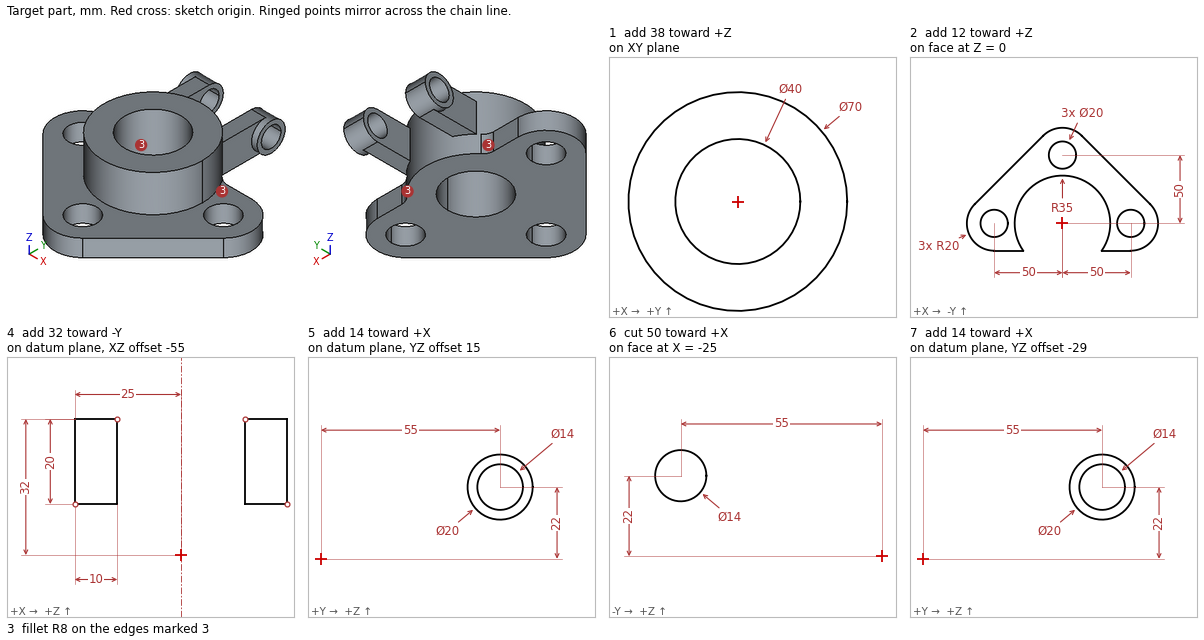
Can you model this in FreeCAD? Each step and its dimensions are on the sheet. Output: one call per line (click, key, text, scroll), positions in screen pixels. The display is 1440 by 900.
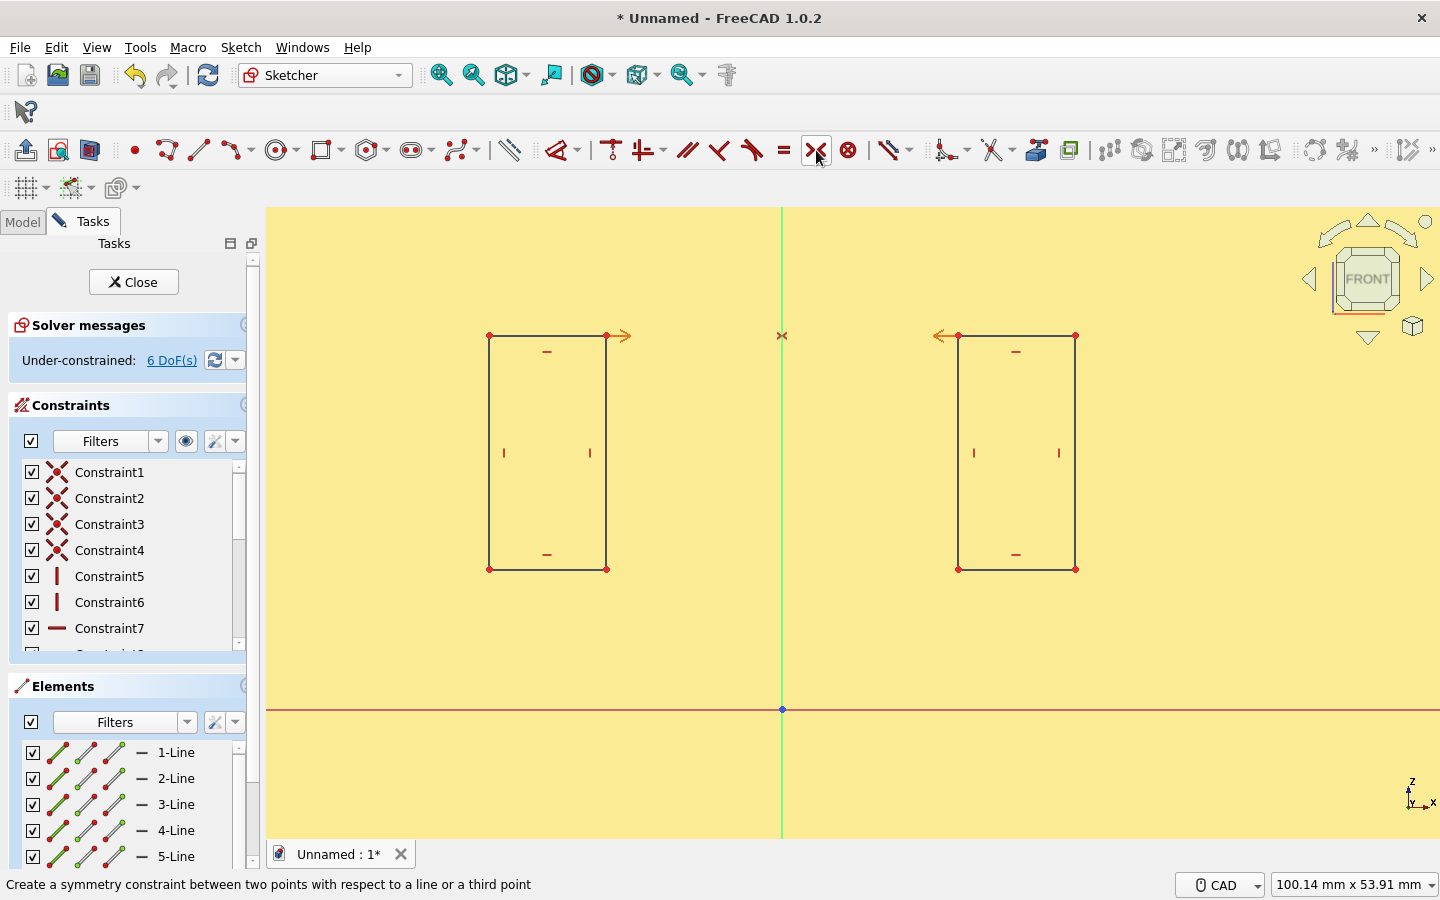
click(489, 570)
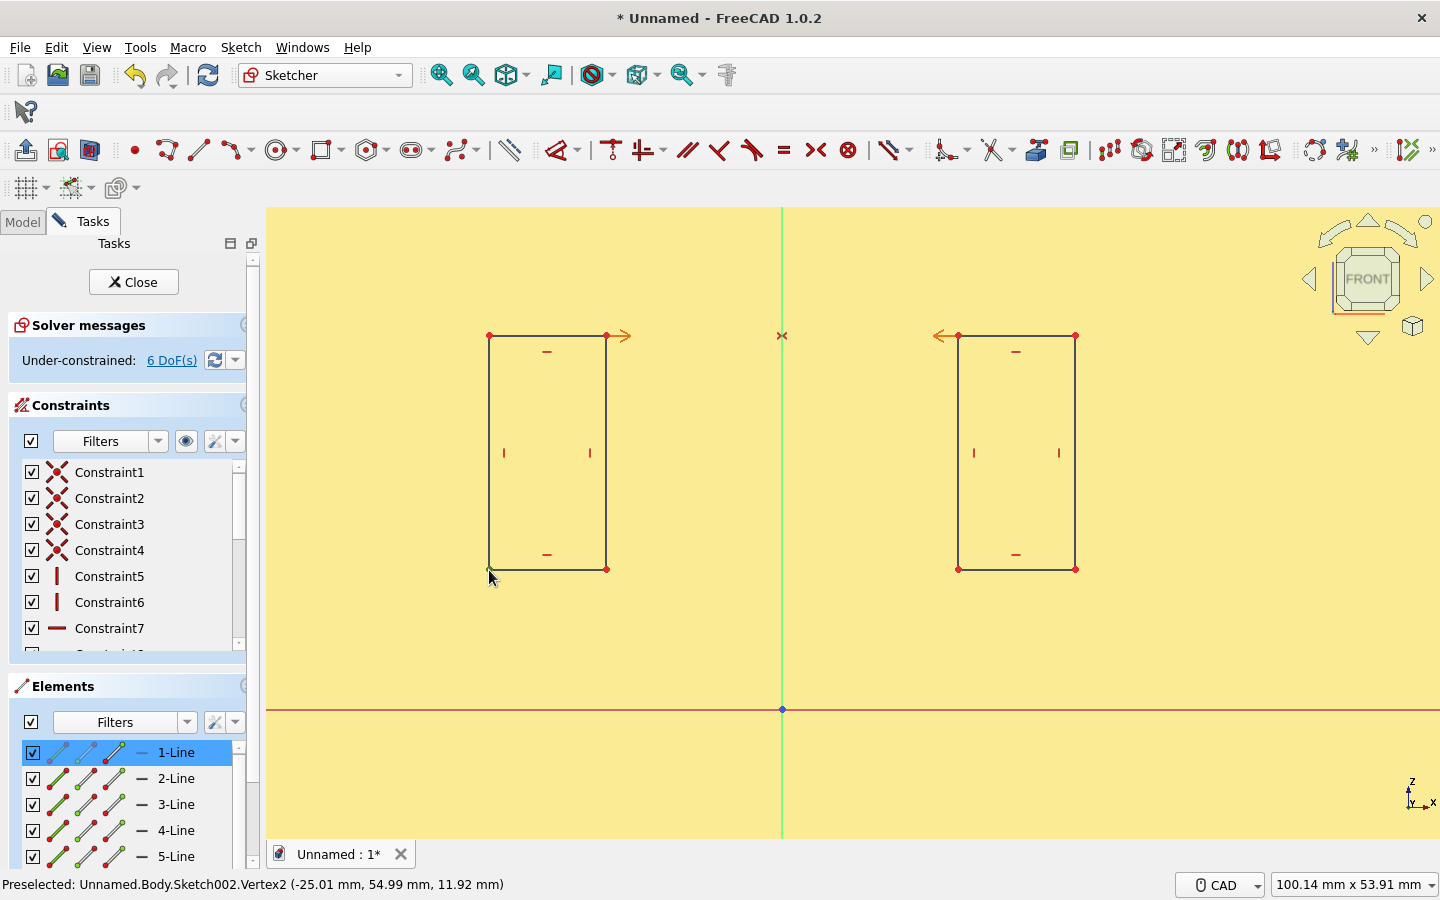
click(1075, 570)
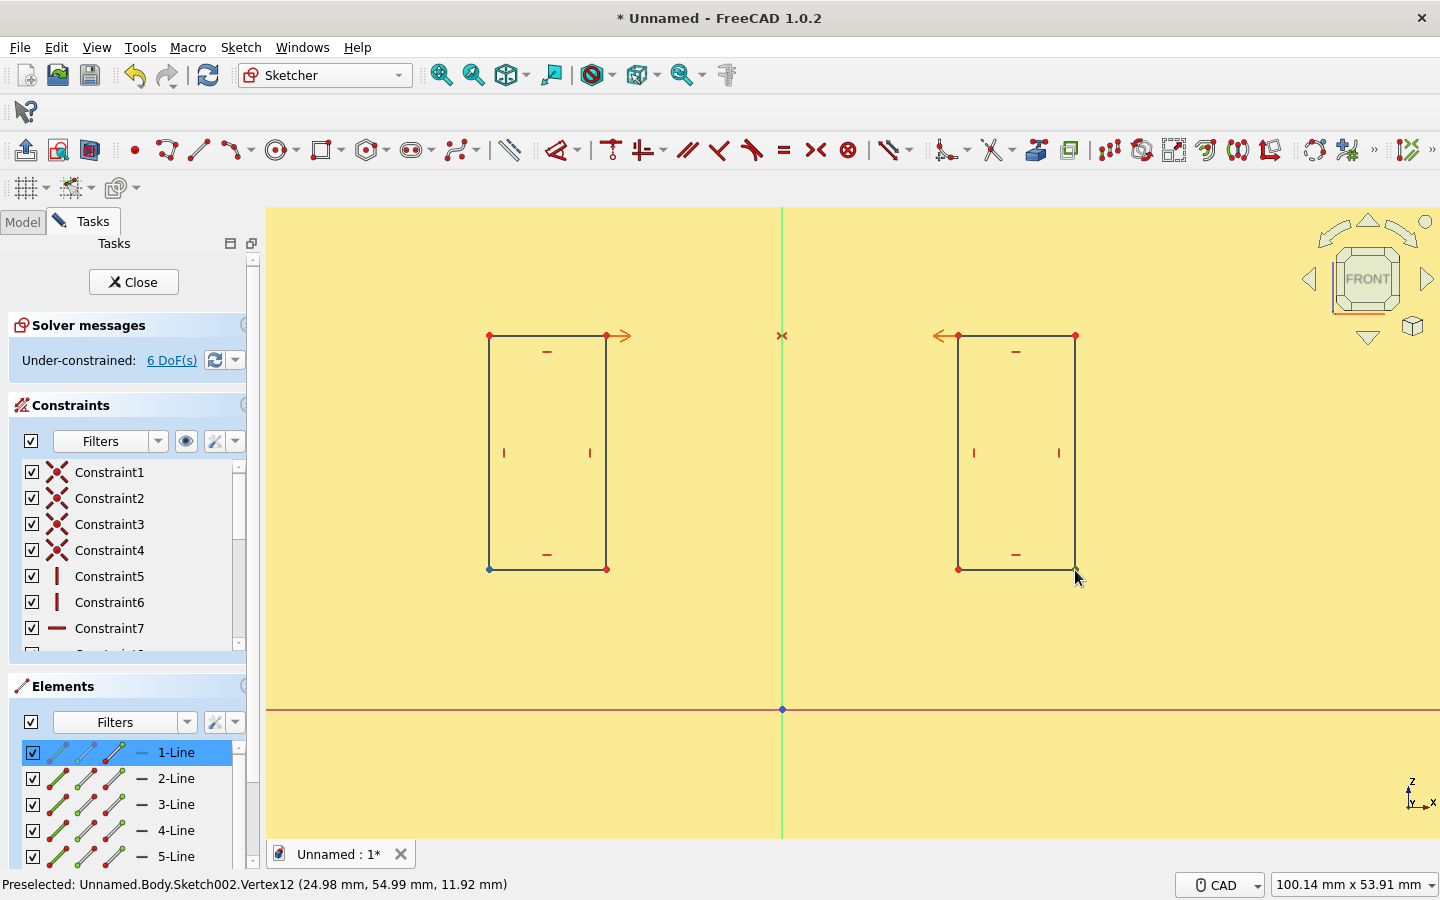
click(782, 770)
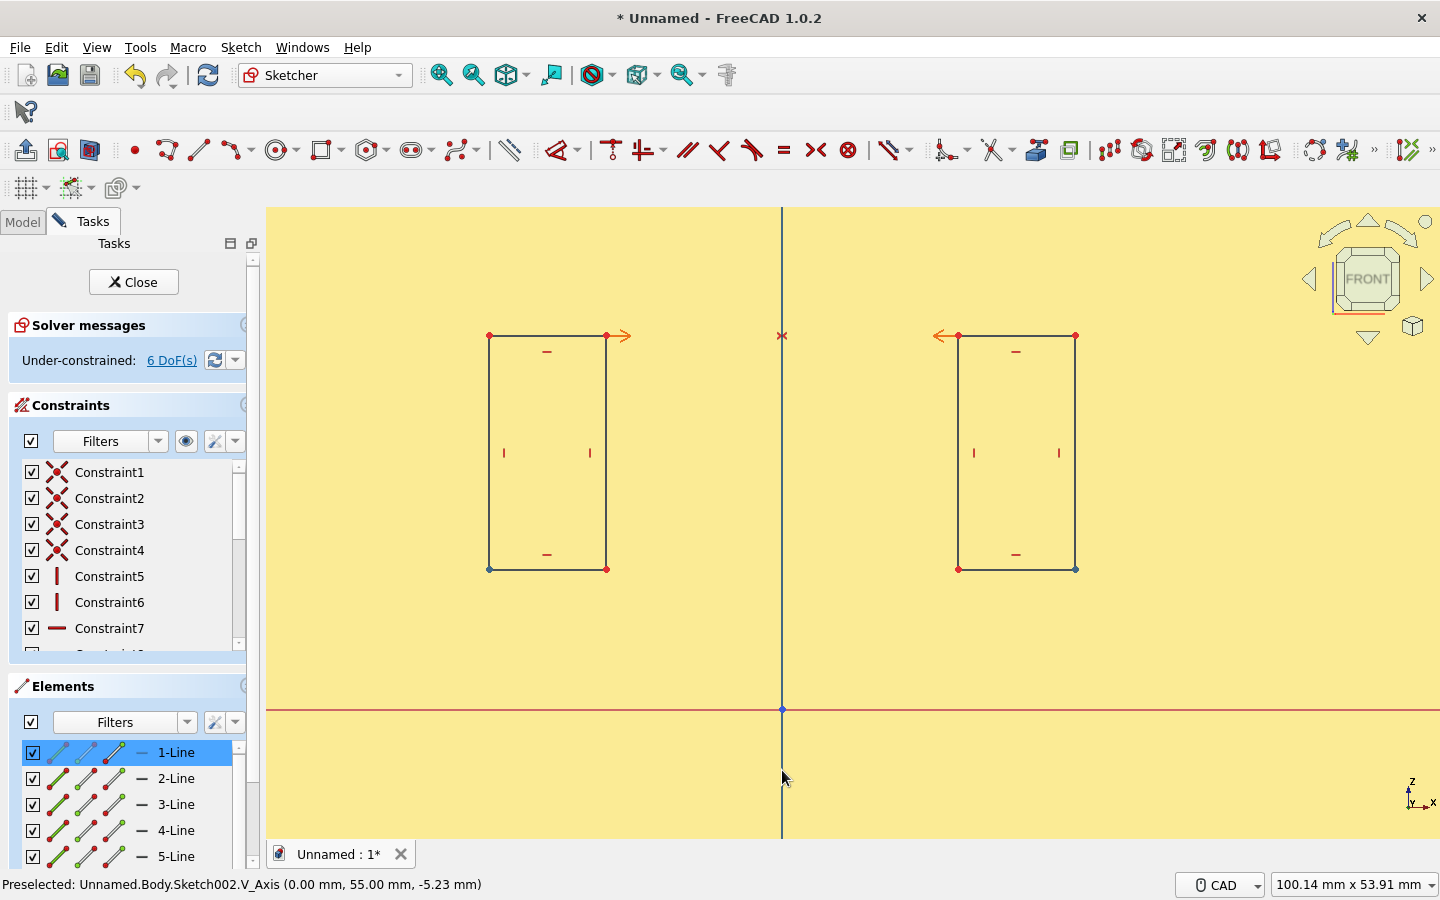
key(s)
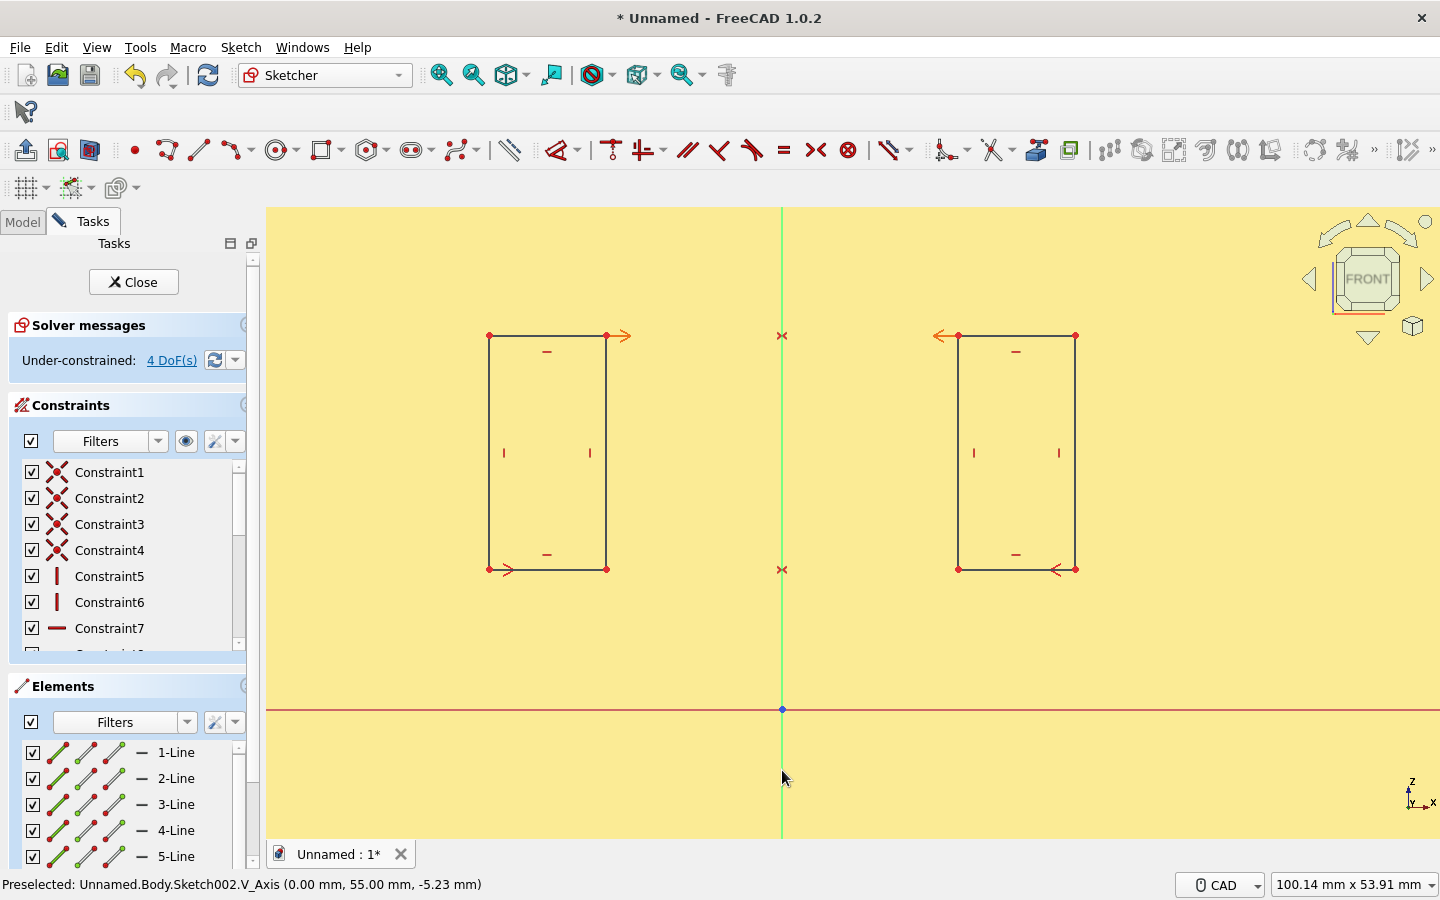
key(d)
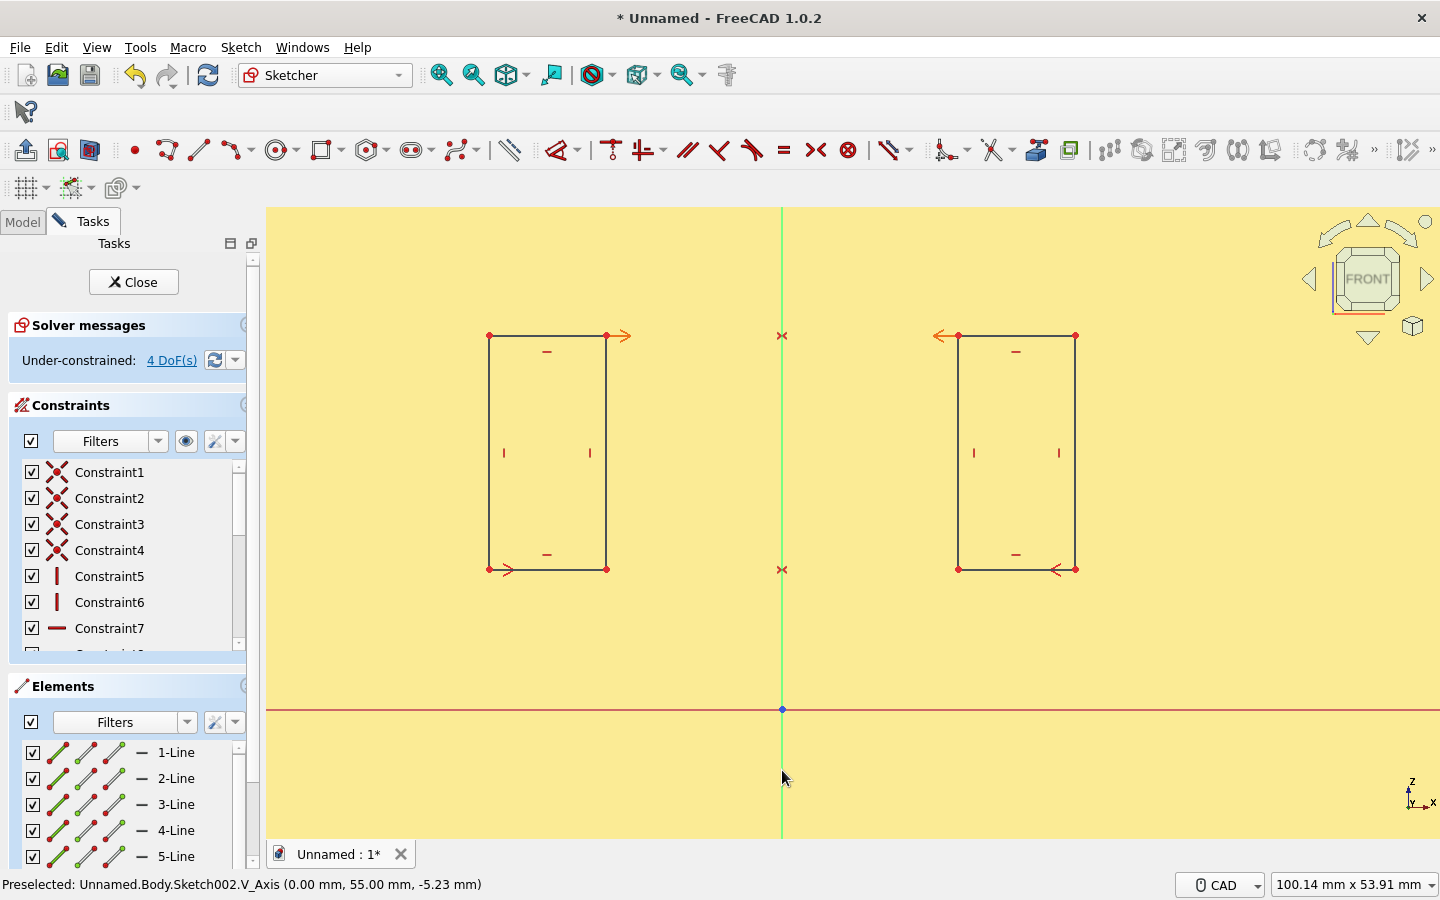
click(489, 406)
click(455, 453)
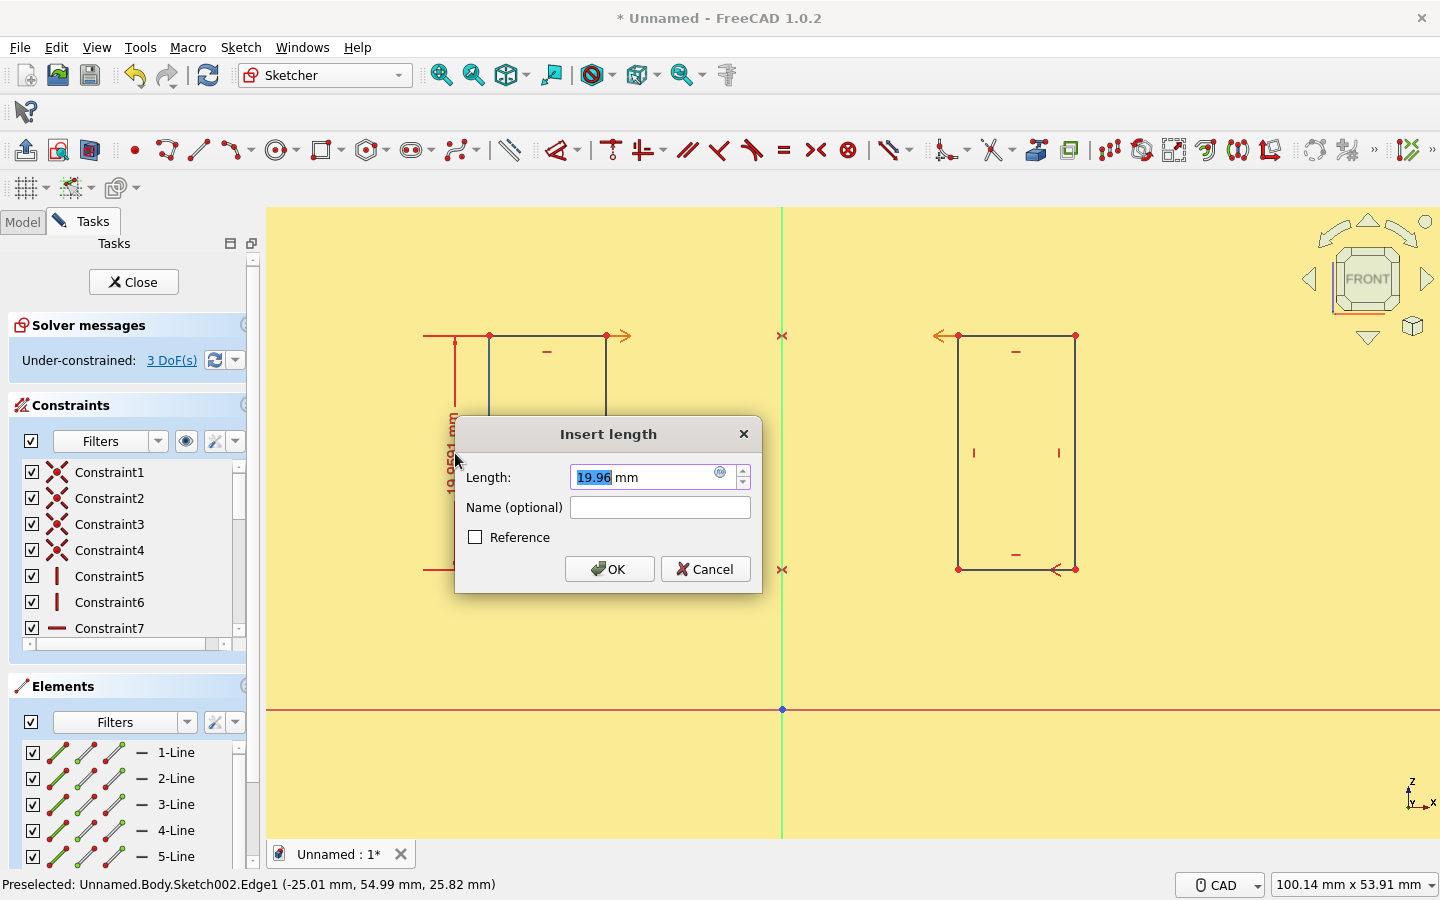
text(20)
key(Return)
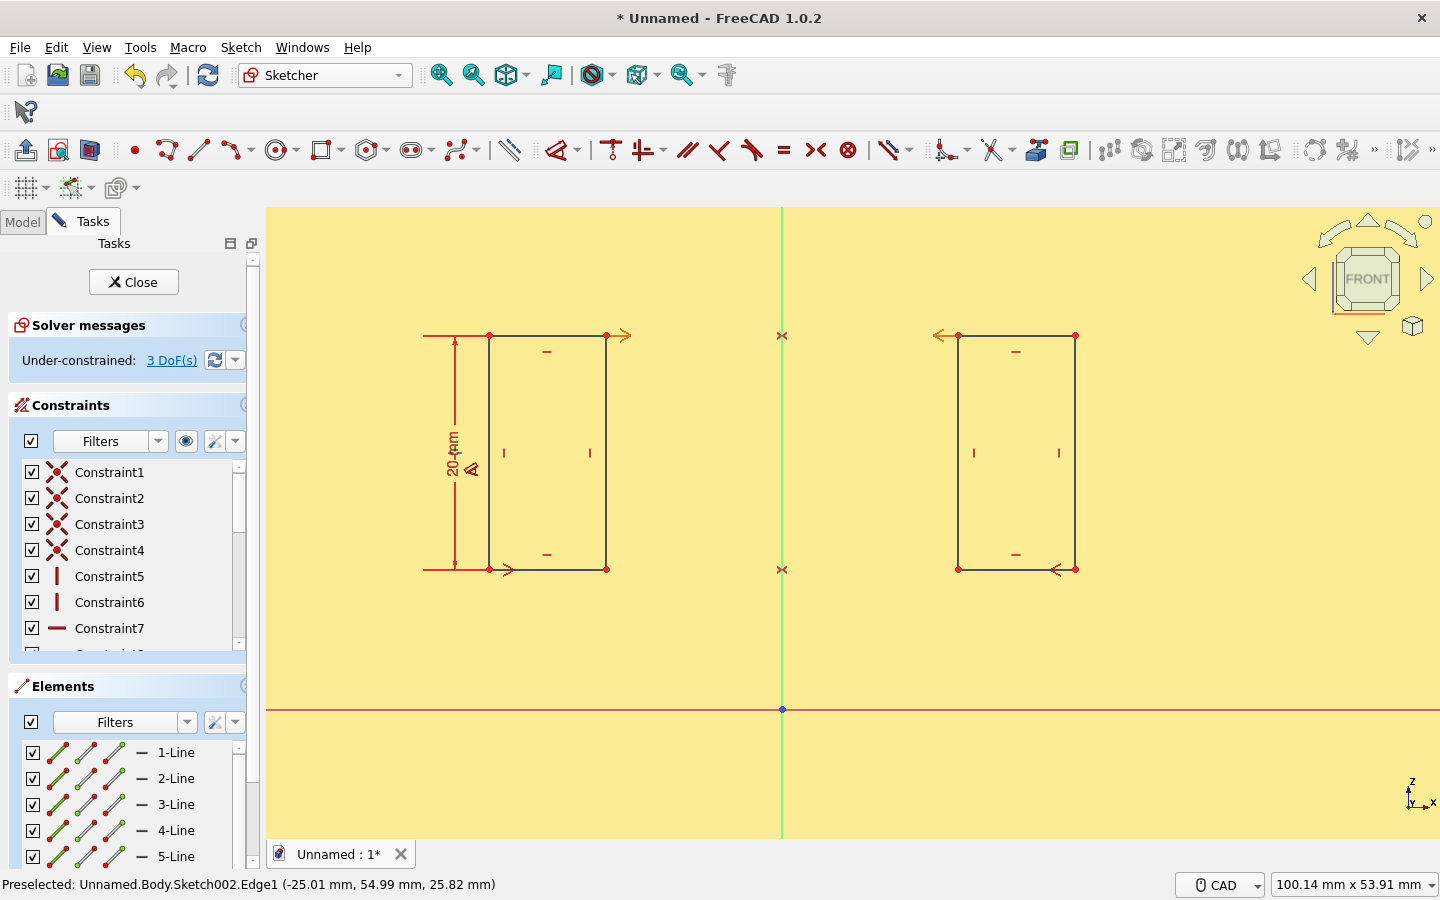
click(524, 570)
click(547, 604)